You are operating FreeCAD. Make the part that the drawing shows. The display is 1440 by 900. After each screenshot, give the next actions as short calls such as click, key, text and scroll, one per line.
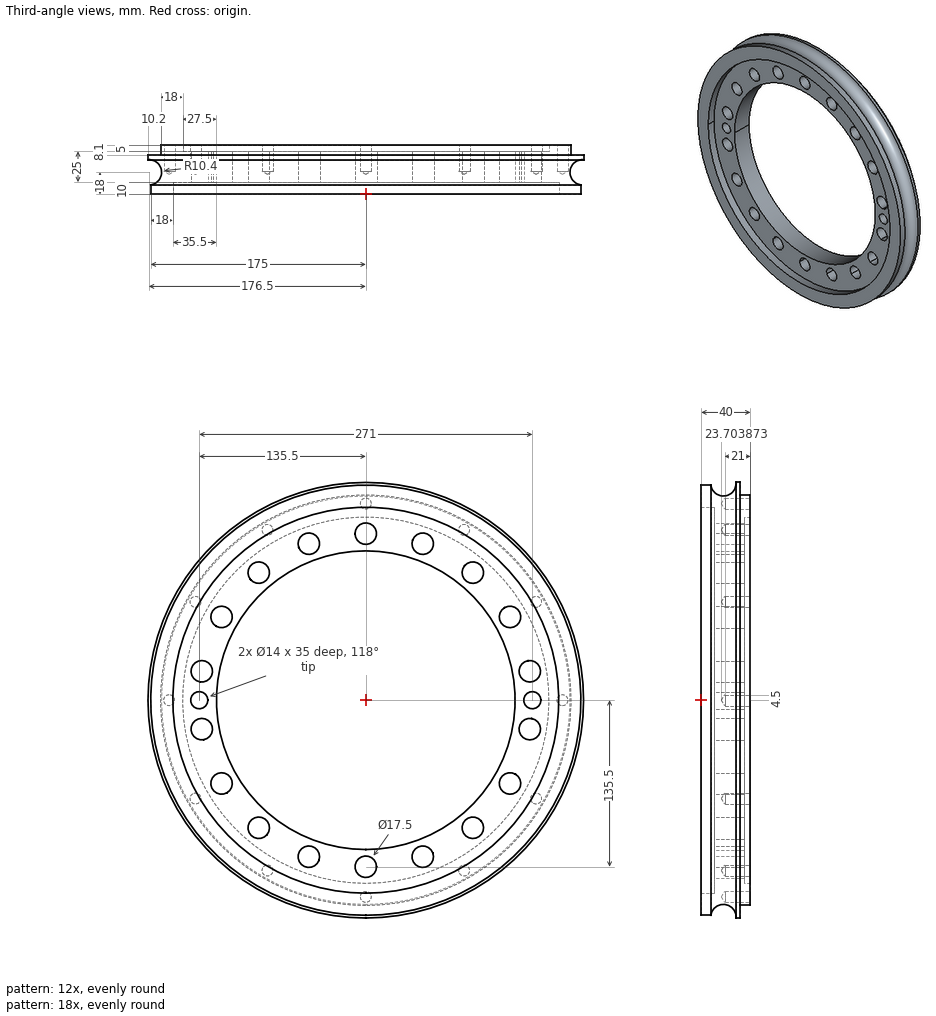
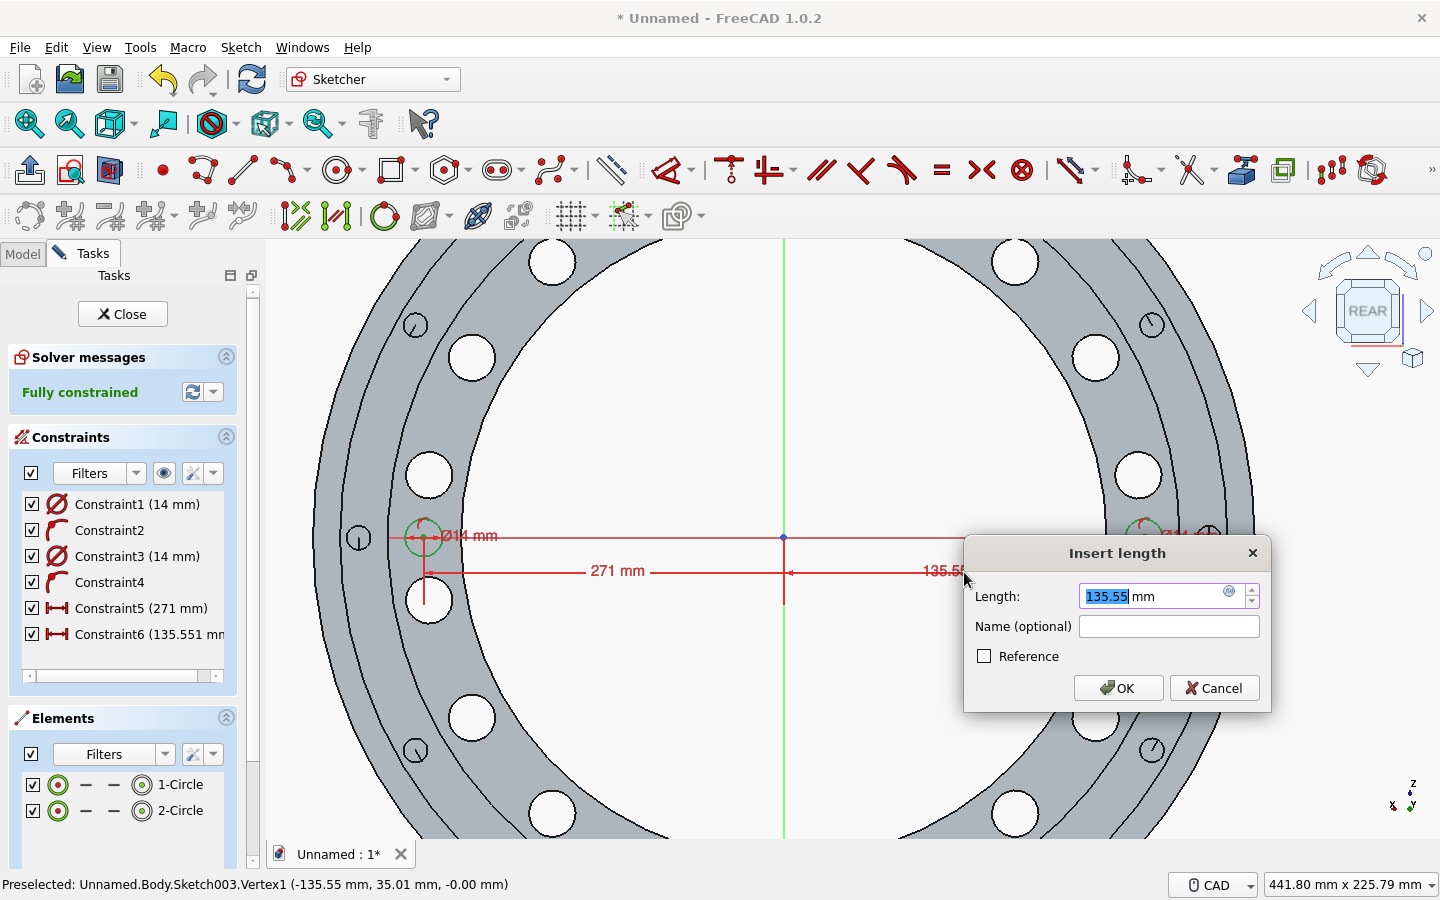
text(135.5)
key(Return)
key(Escape)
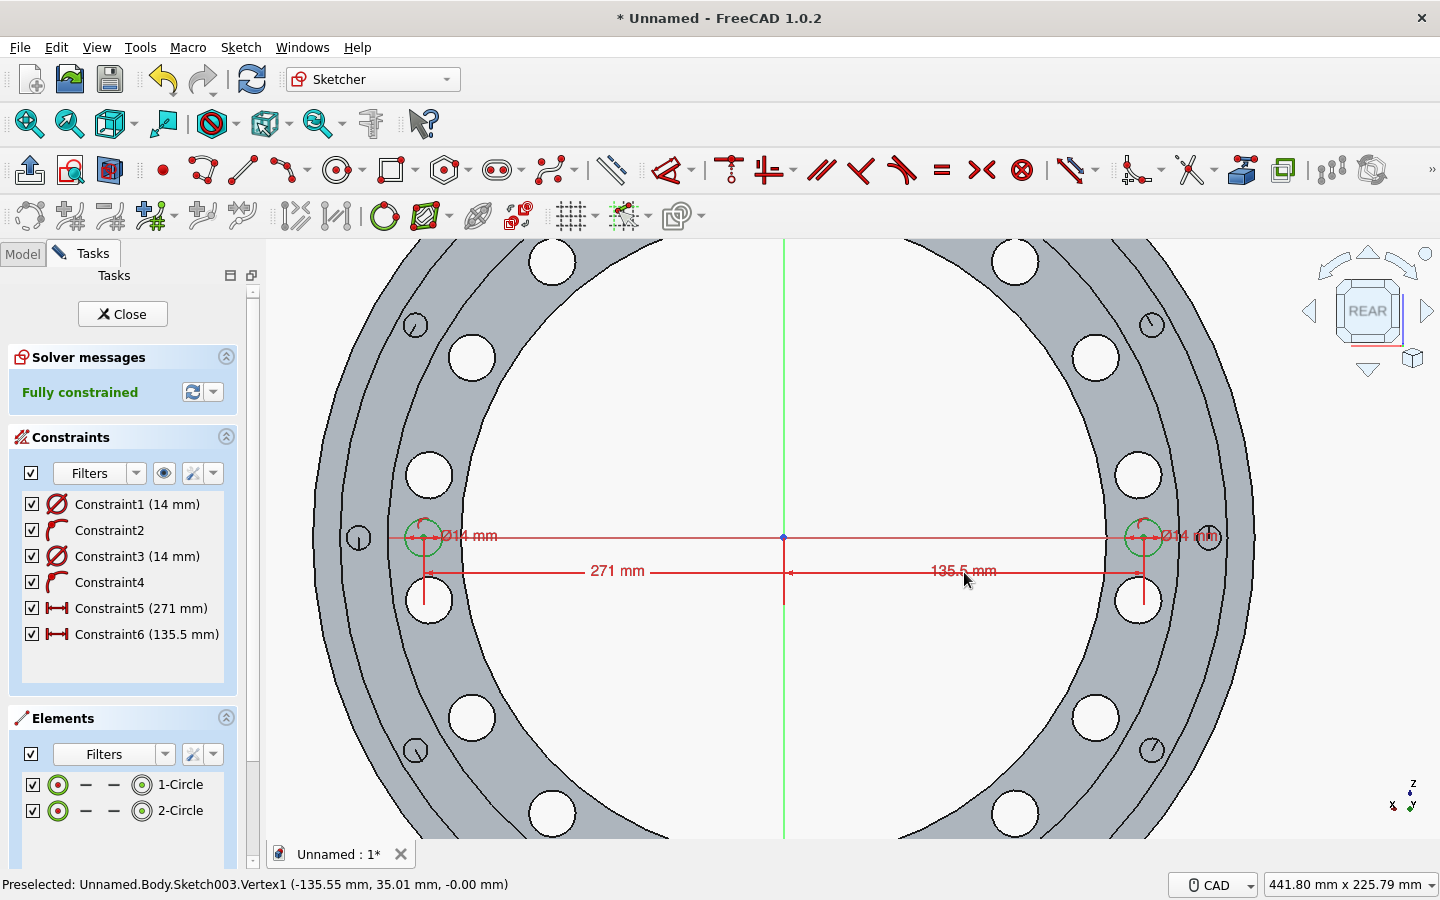
click(123, 314)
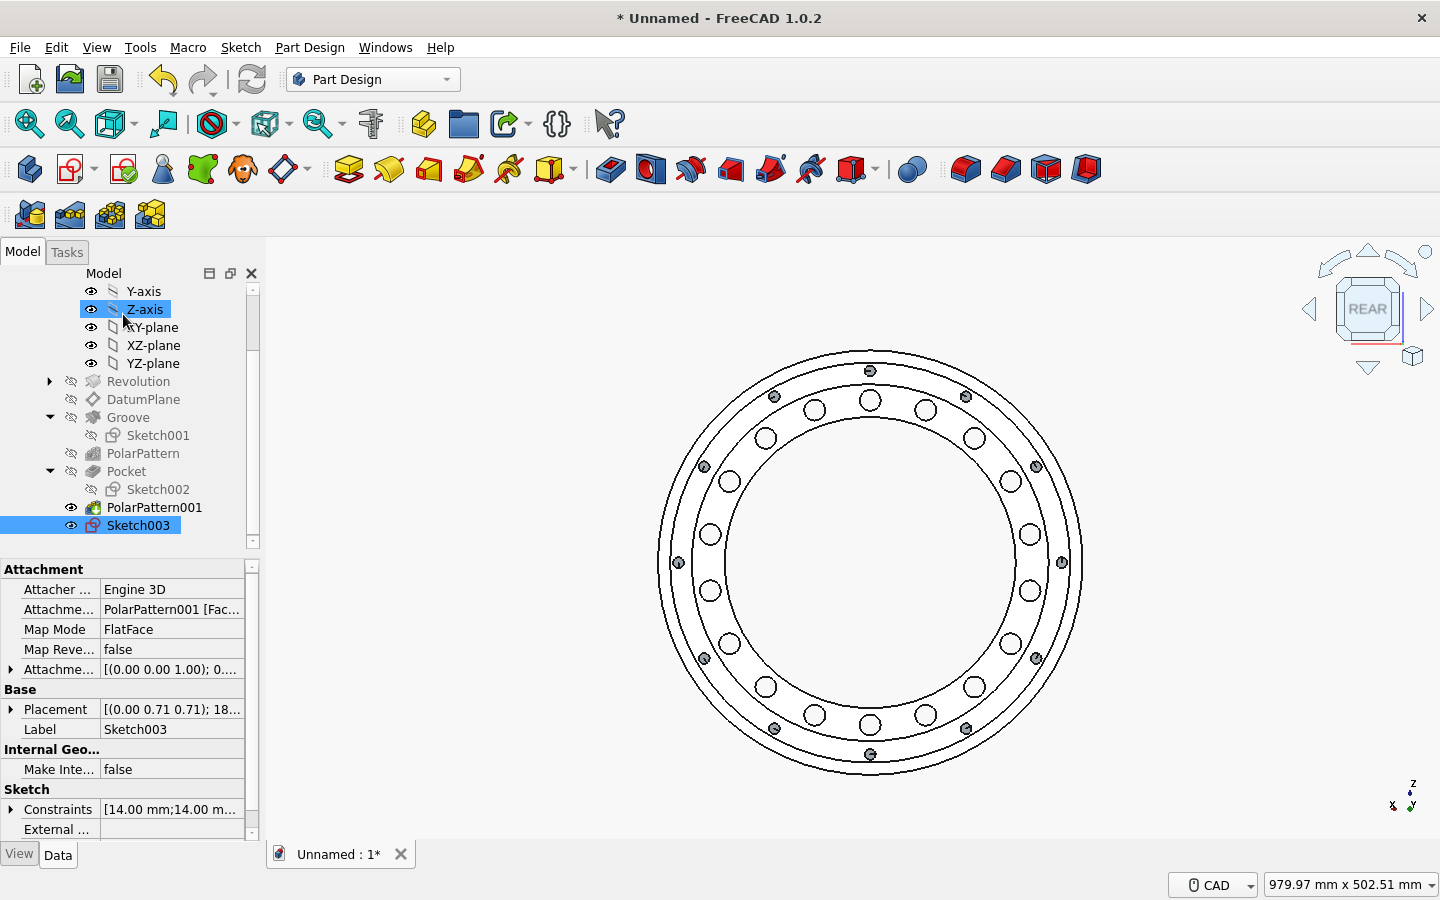
click(652, 170)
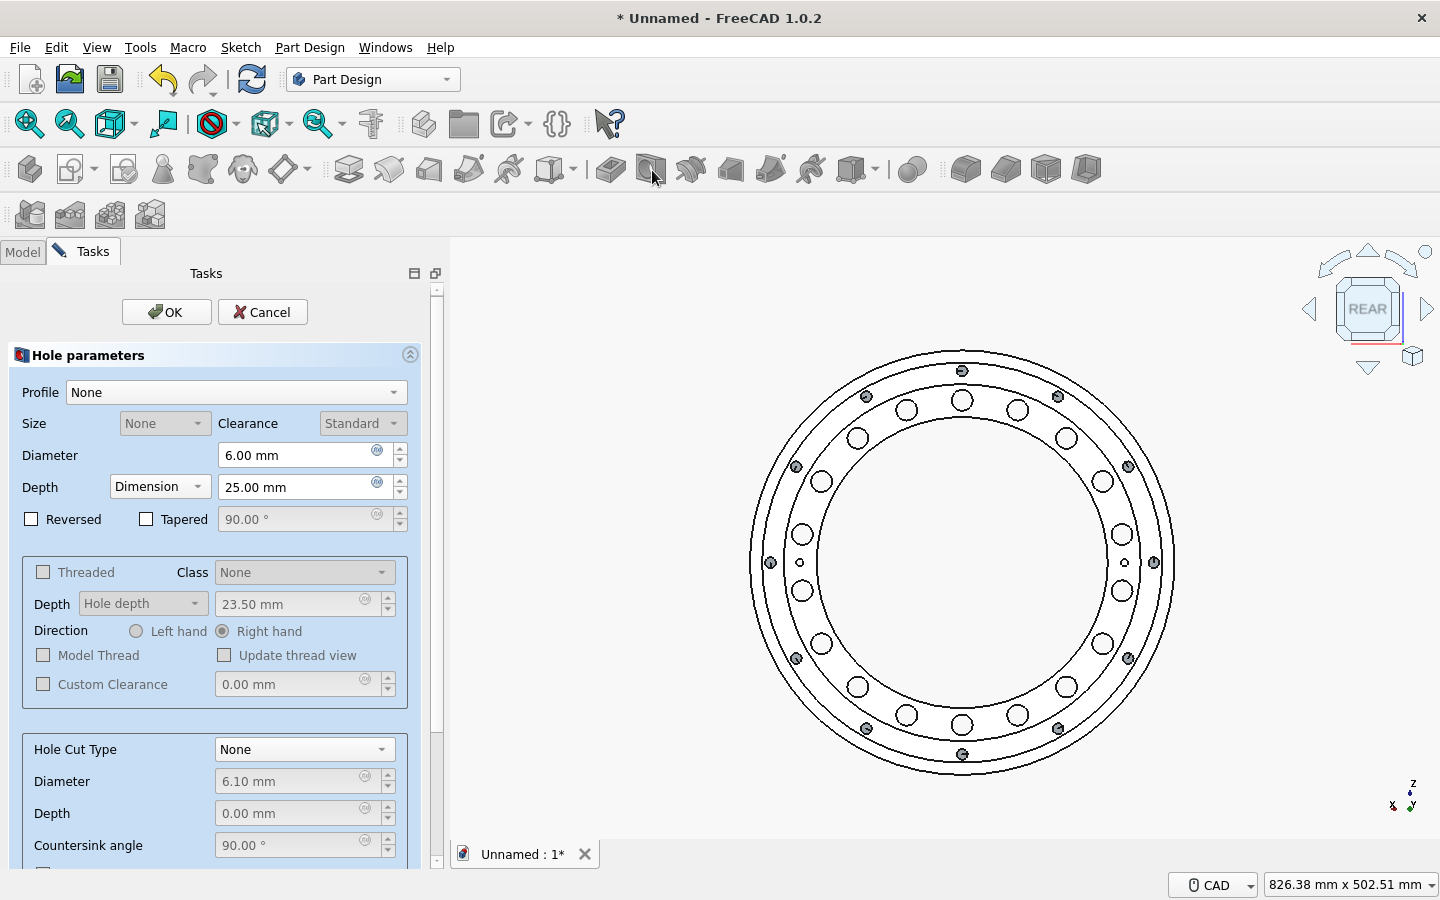
triple_click(305, 455)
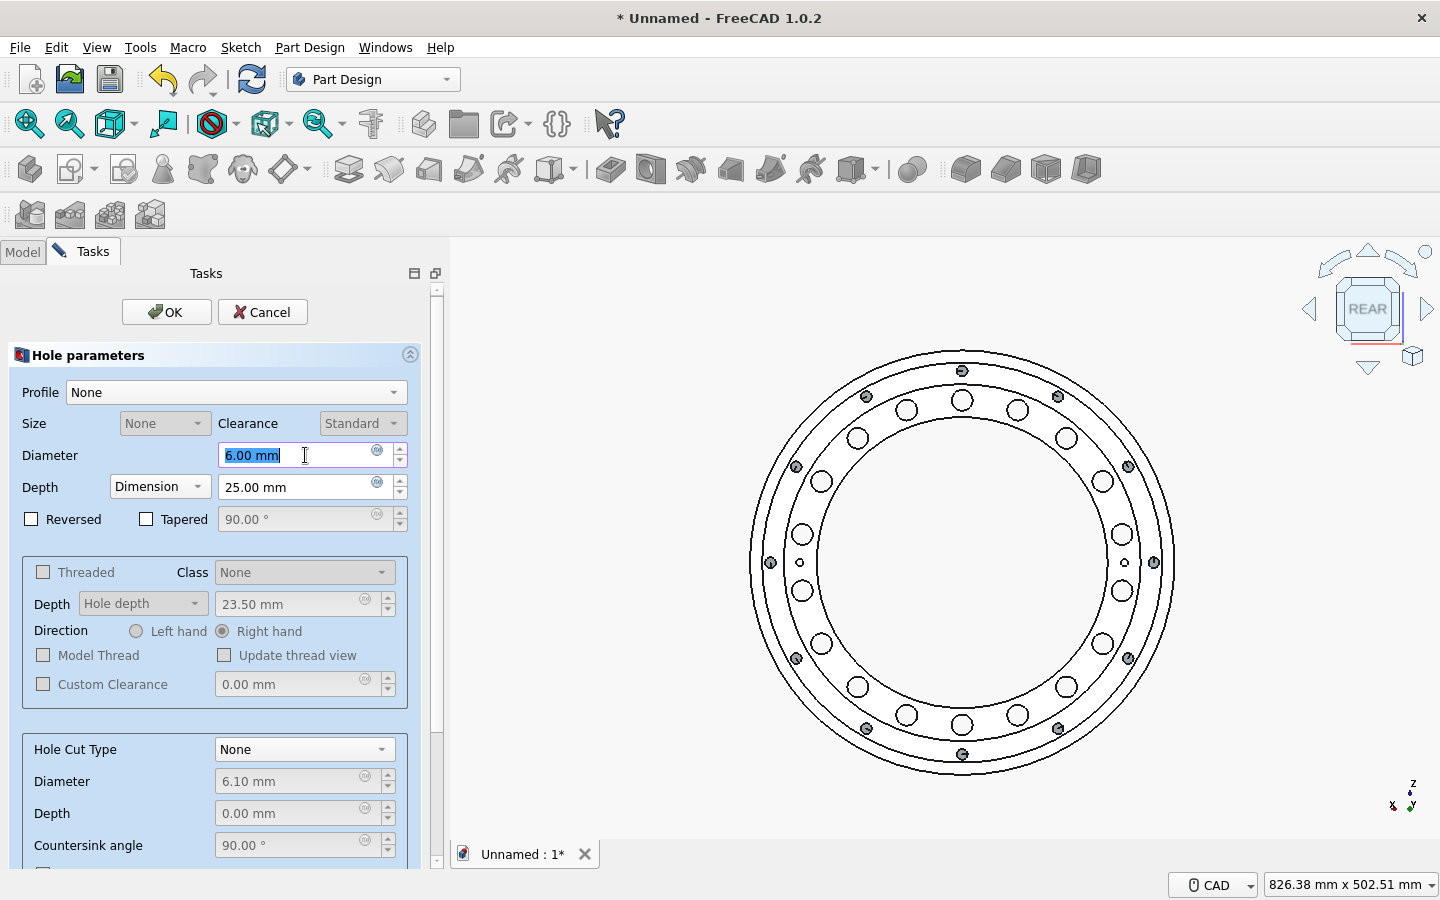
text(14)
key(Tab)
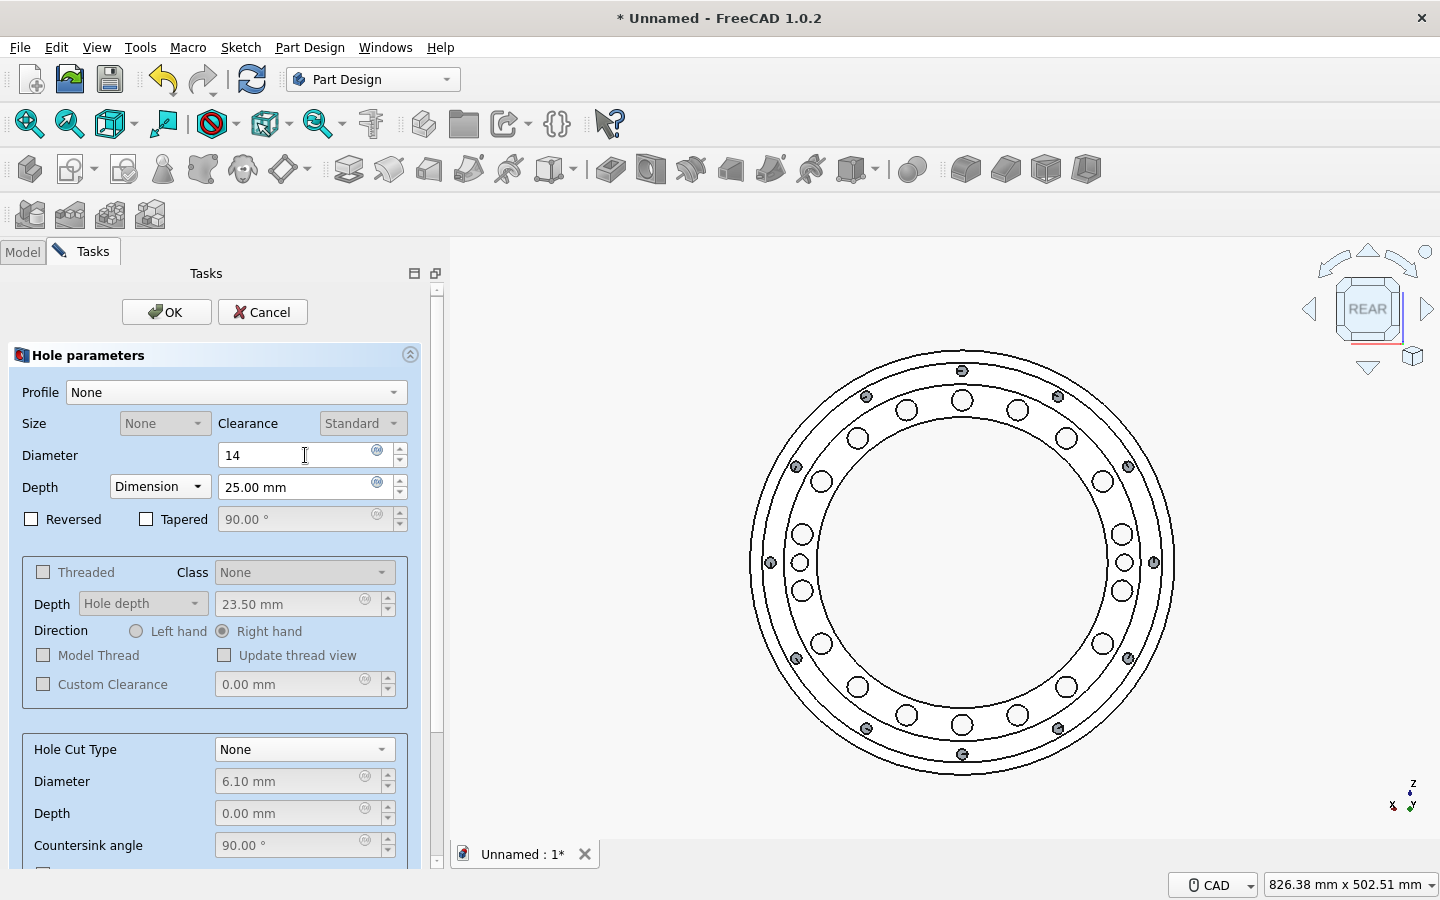
triple_click(305, 487)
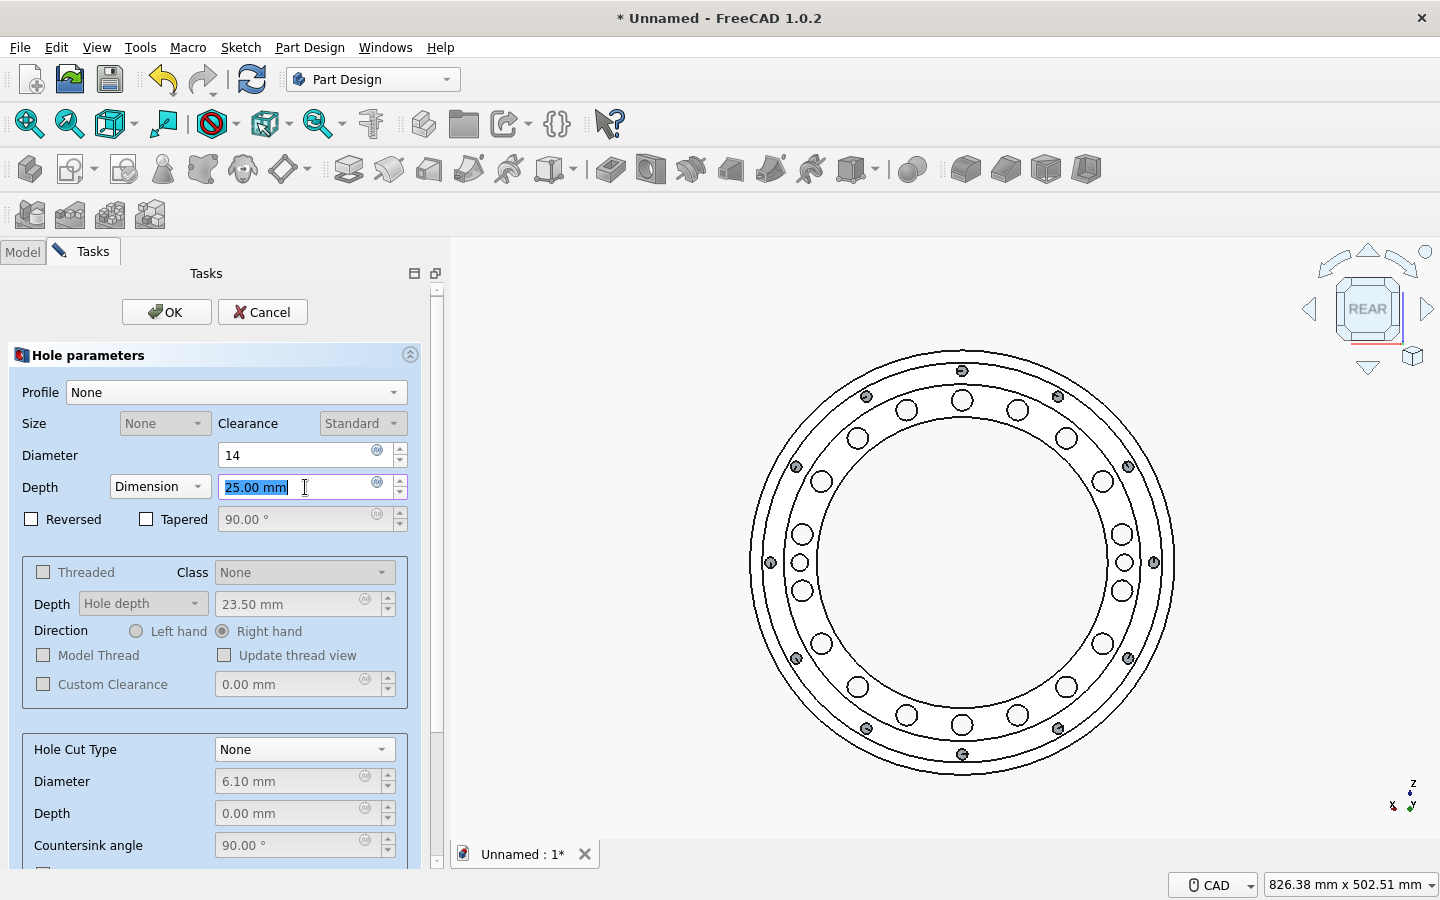
text(35)
key(Tab)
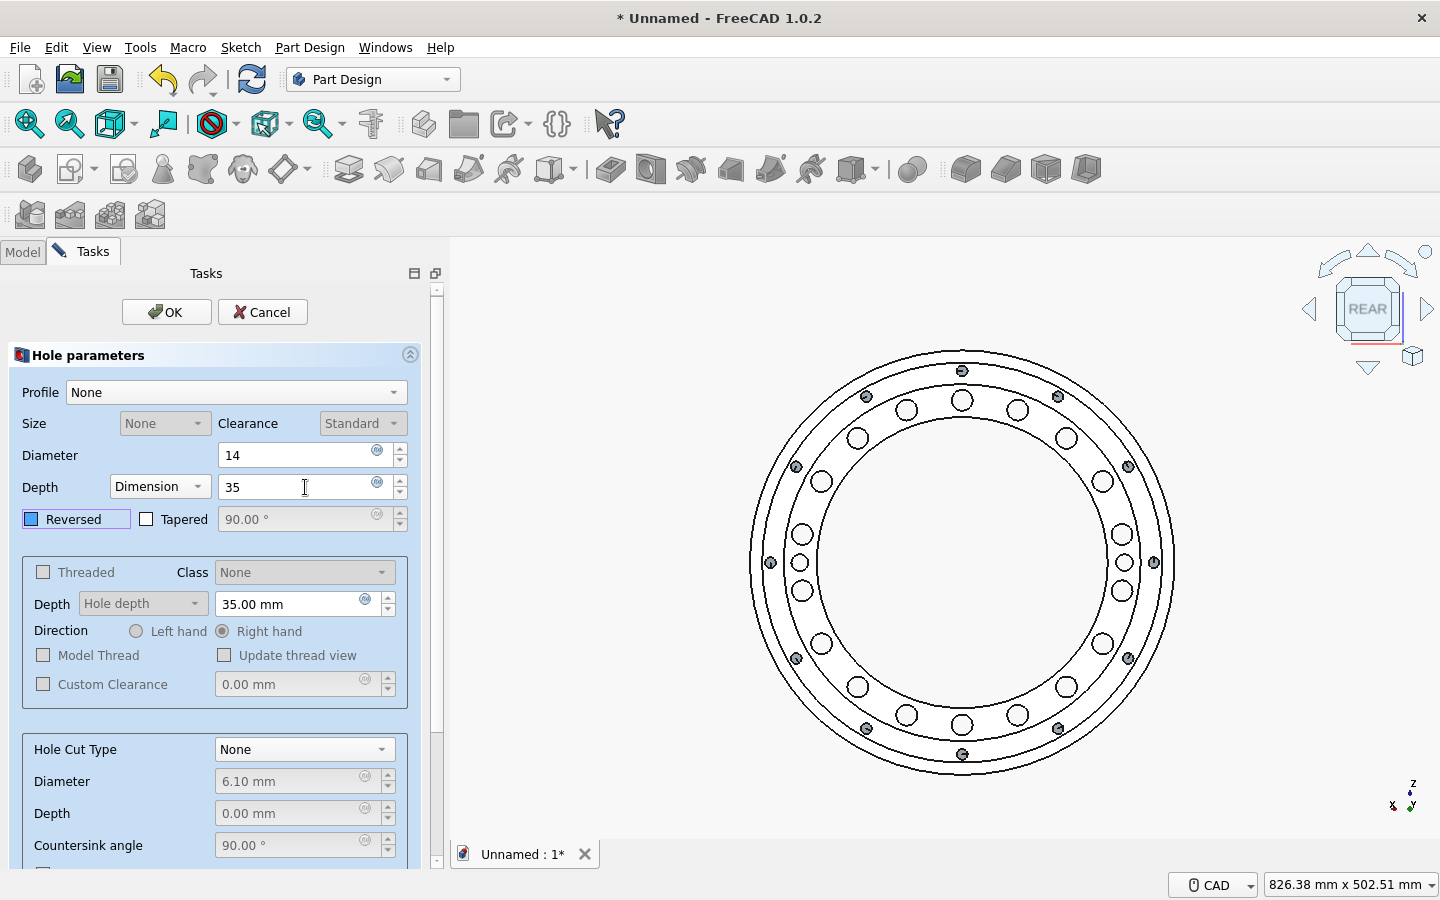
click(167, 312)